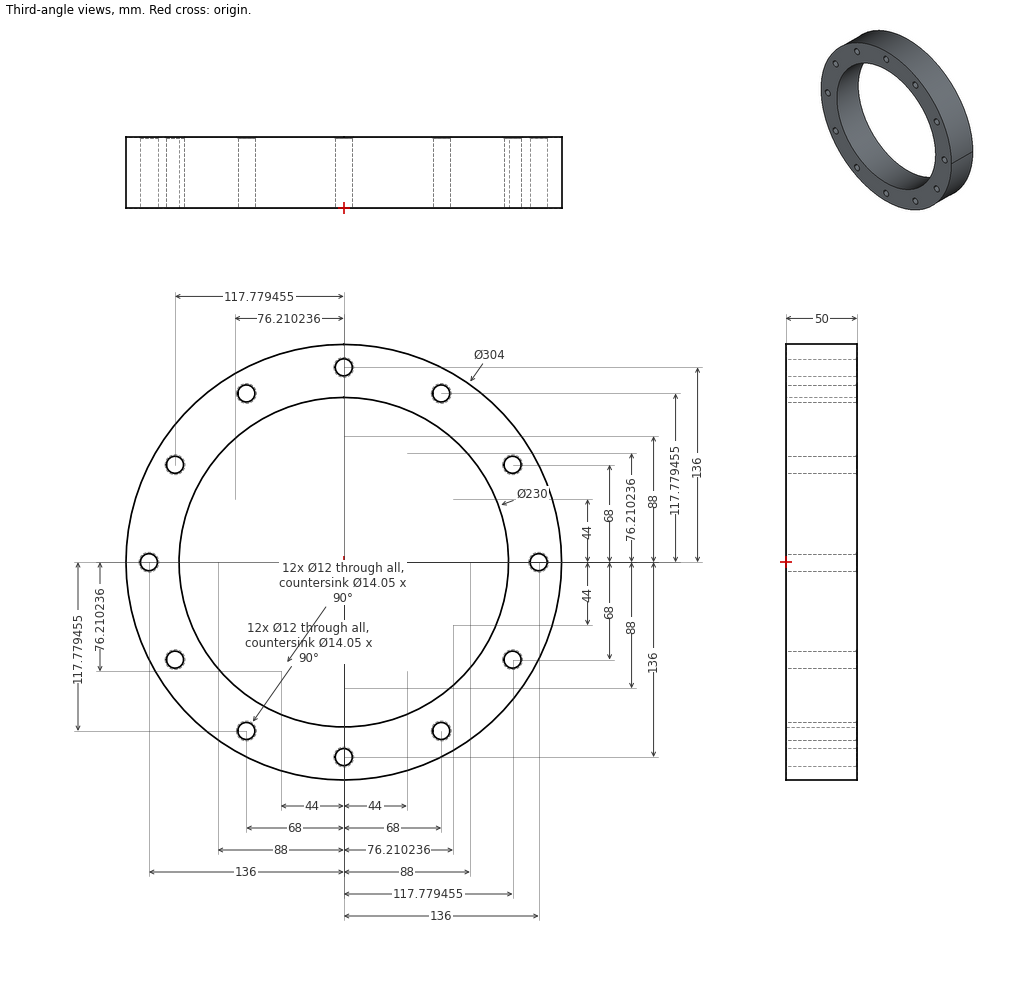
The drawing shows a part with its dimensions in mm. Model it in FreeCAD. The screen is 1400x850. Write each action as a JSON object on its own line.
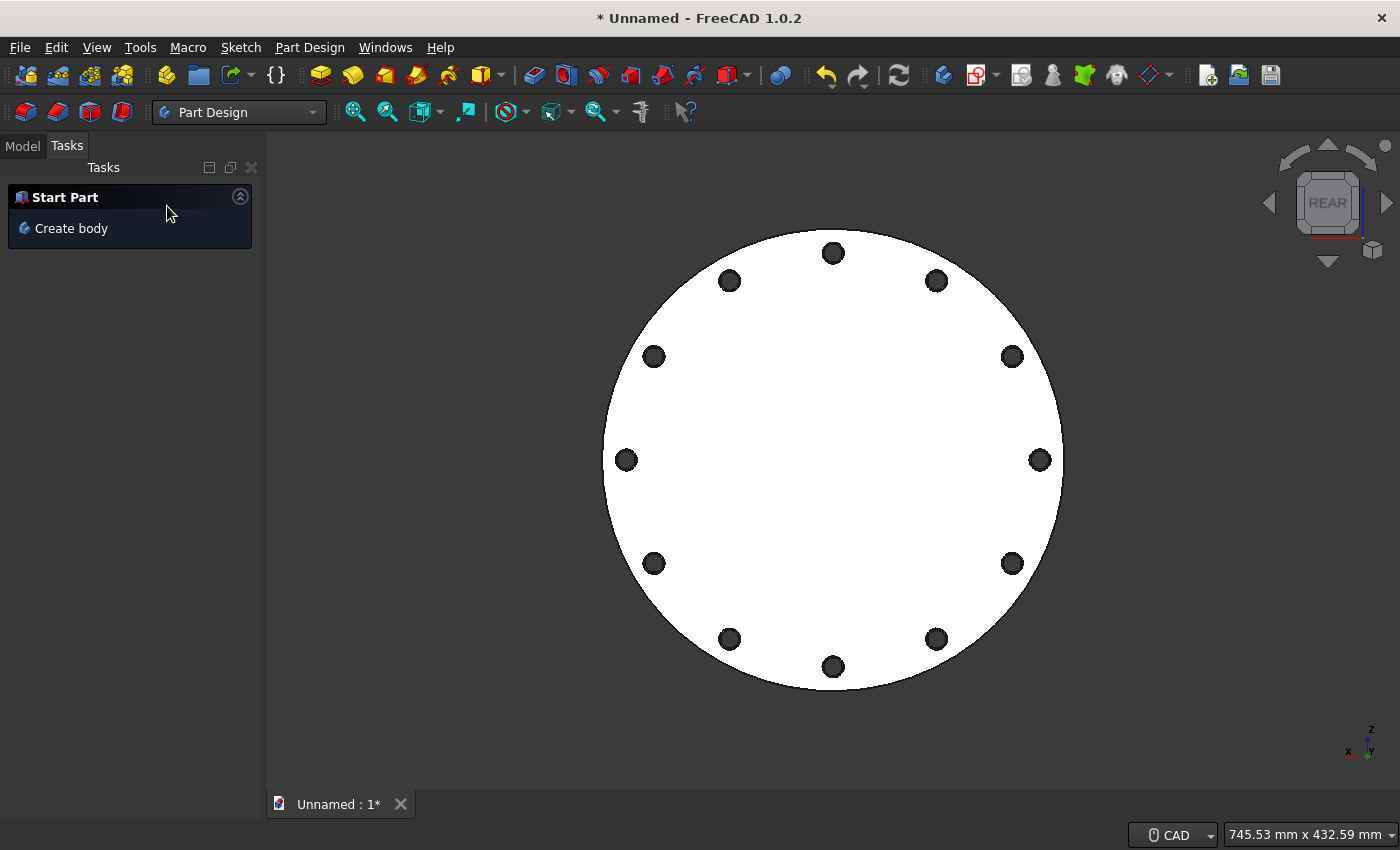
{"action": "left_click", "coordinate": [833, 459]}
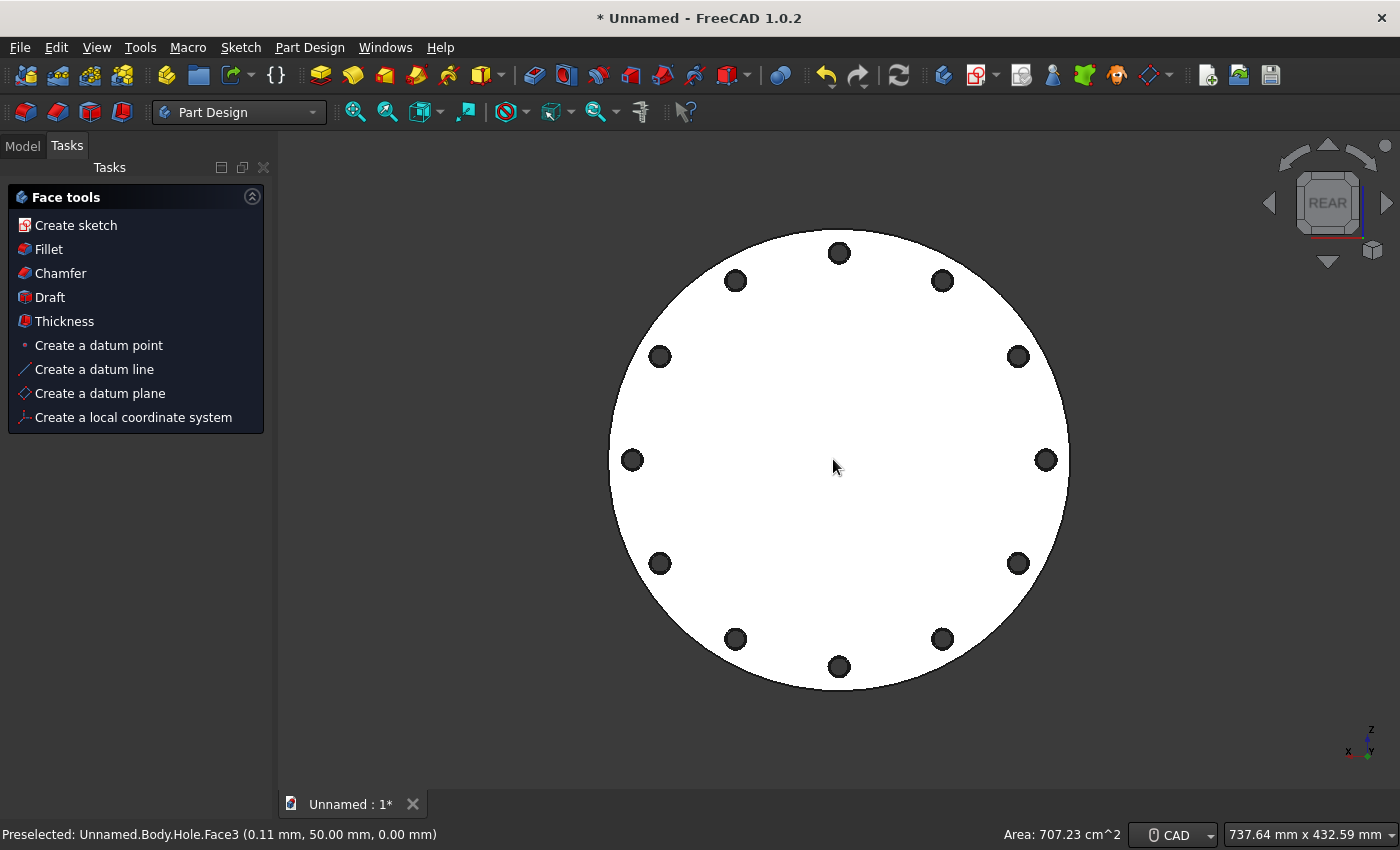
{"action": "left_click", "coordinate": [976, 76]}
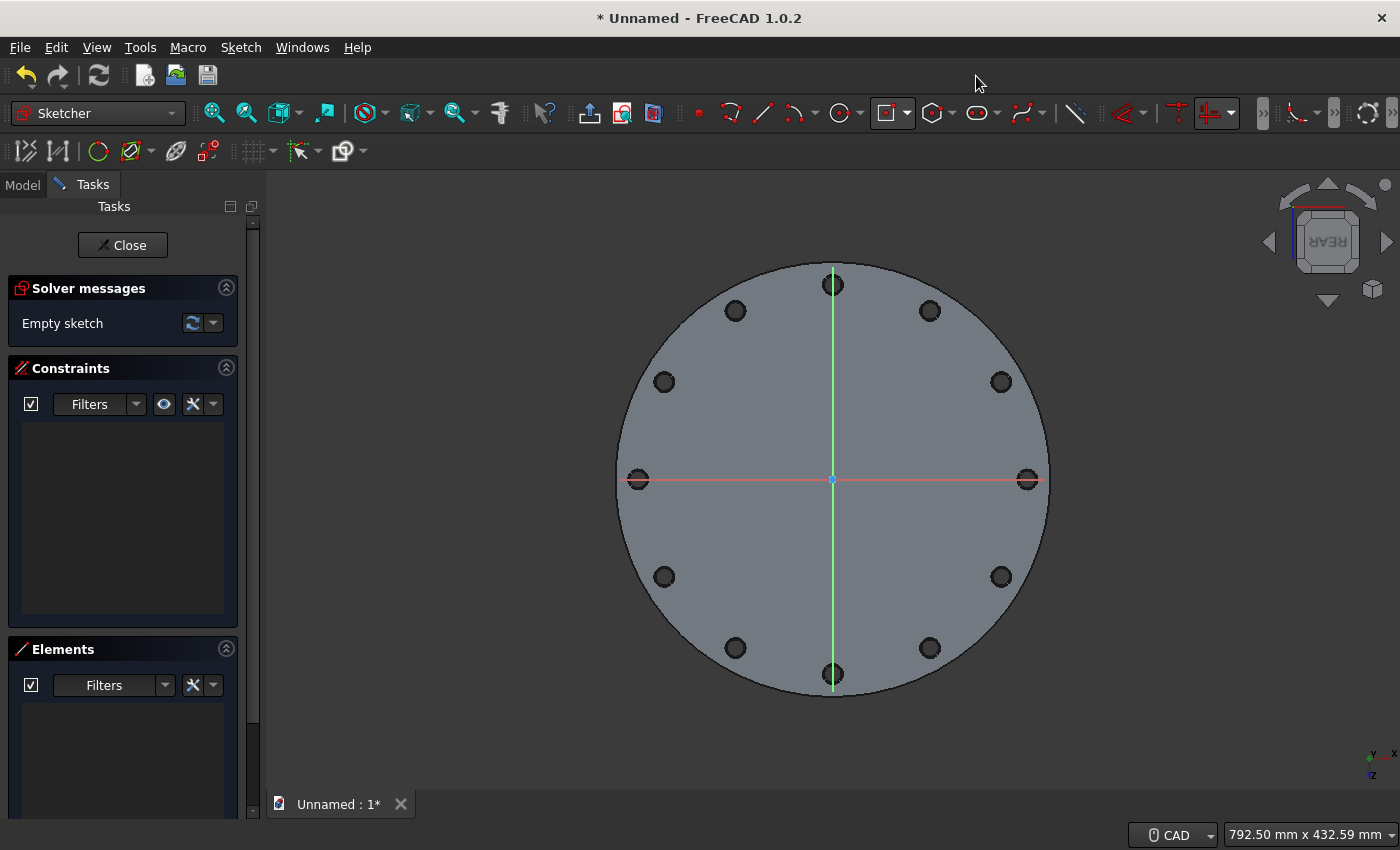
{"action": "left_click", "coordinate": [840, 114]}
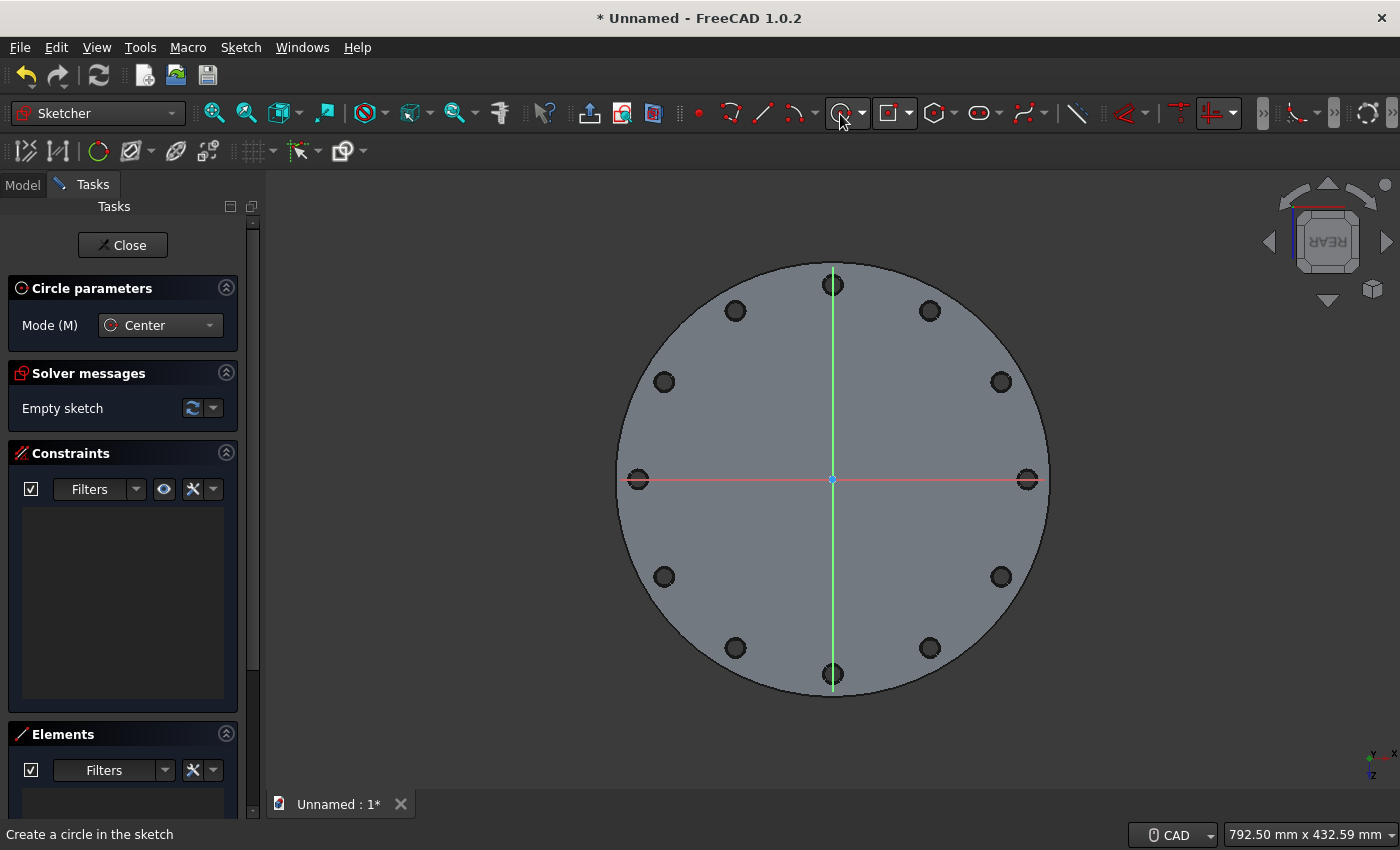
{"action": "left_click", "coordinate": [833, 479]}
{"action": "left_click", "coordinate": [949, 363]}
{"action": "key", "text": "Escape"}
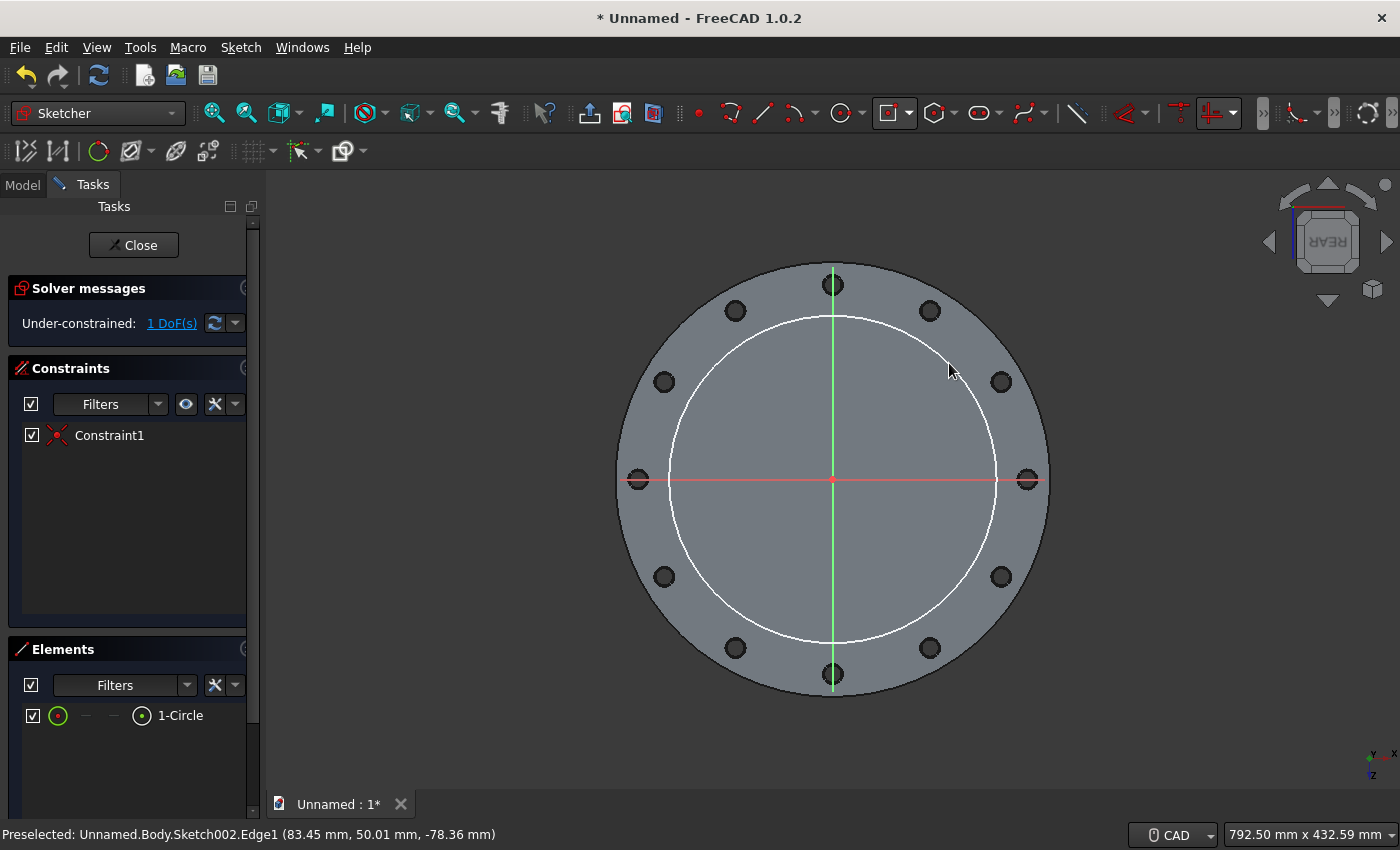
{"action": "key", "text": "d"}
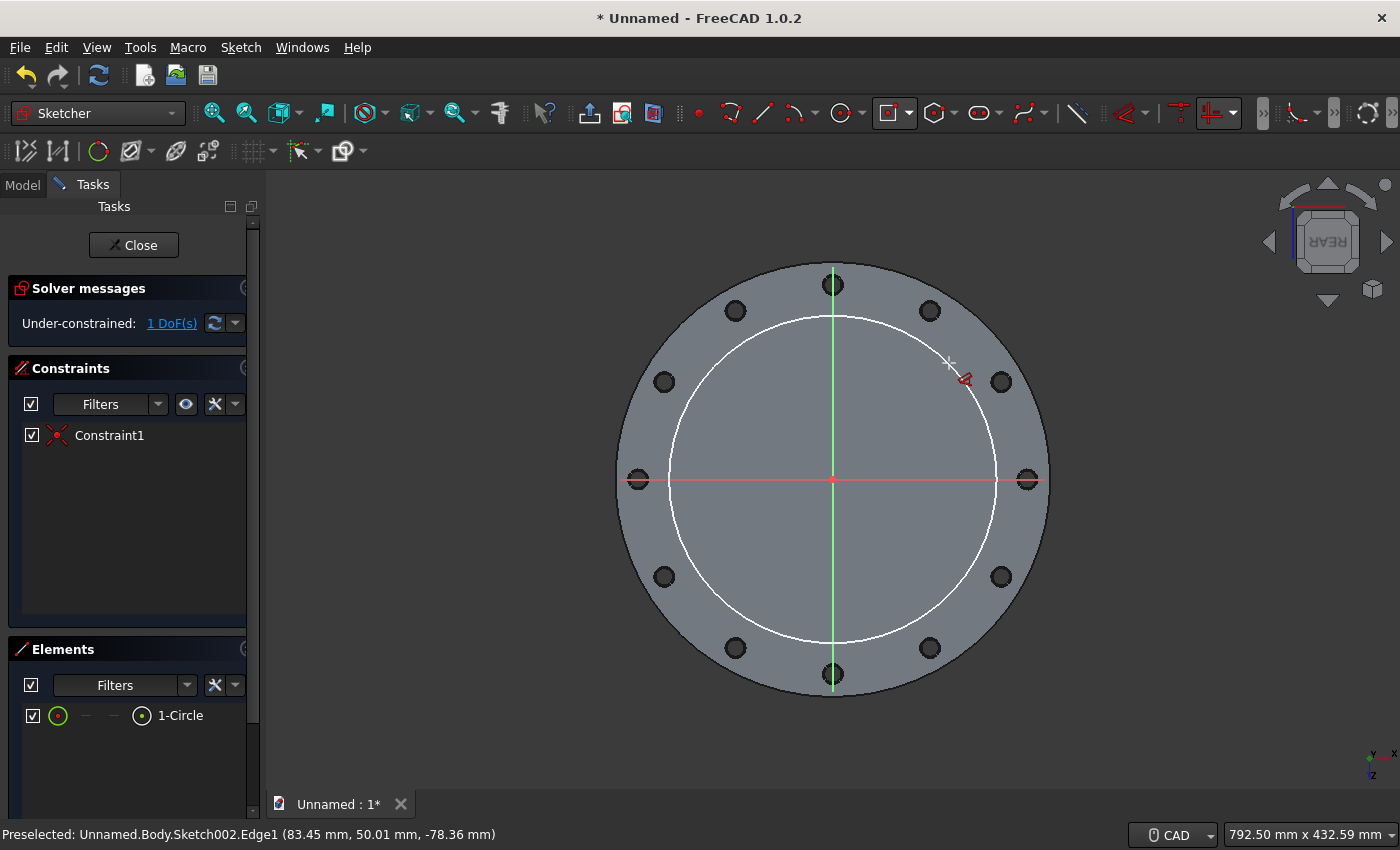
{"action": "left_click", "coordinate": [948, 363]}
{"action": "left_click", "coordinate": [970, 340]}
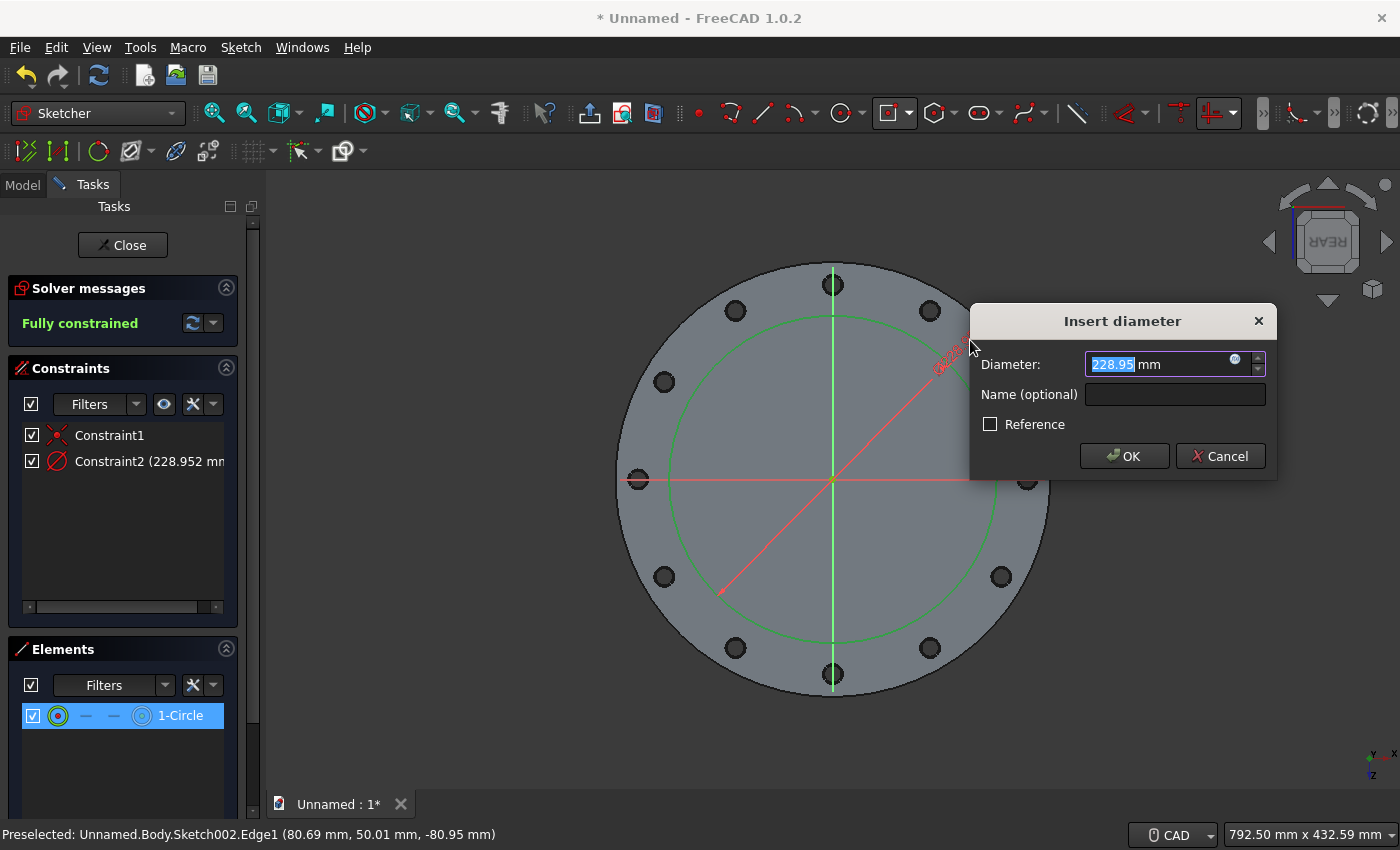
{"action": "type", "text": "230"}
{"action": "key", "text": "Return"}
{"action": "key", "text": "Escape"}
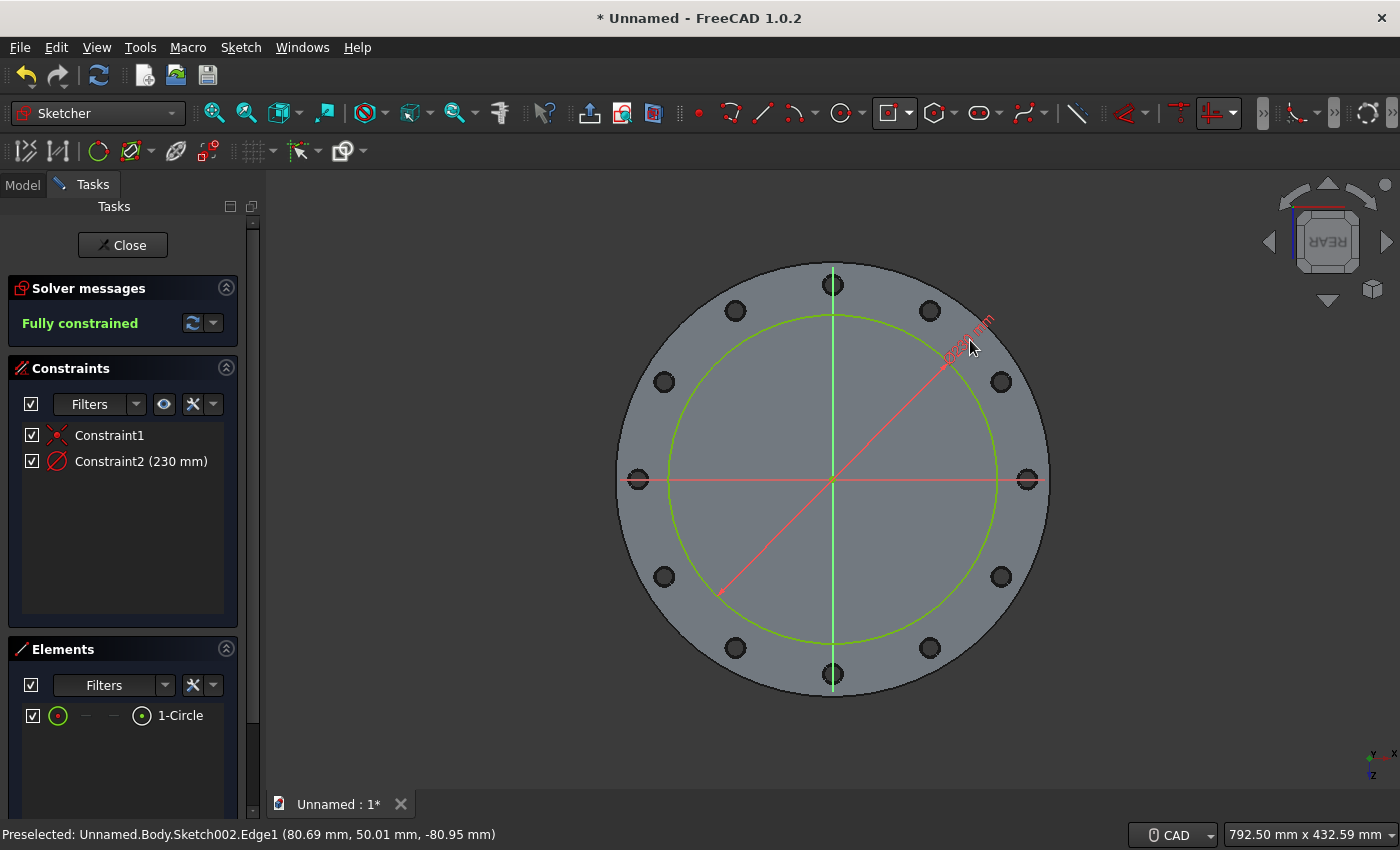
{"action": "left_click", "coordinate": [123, 245]}